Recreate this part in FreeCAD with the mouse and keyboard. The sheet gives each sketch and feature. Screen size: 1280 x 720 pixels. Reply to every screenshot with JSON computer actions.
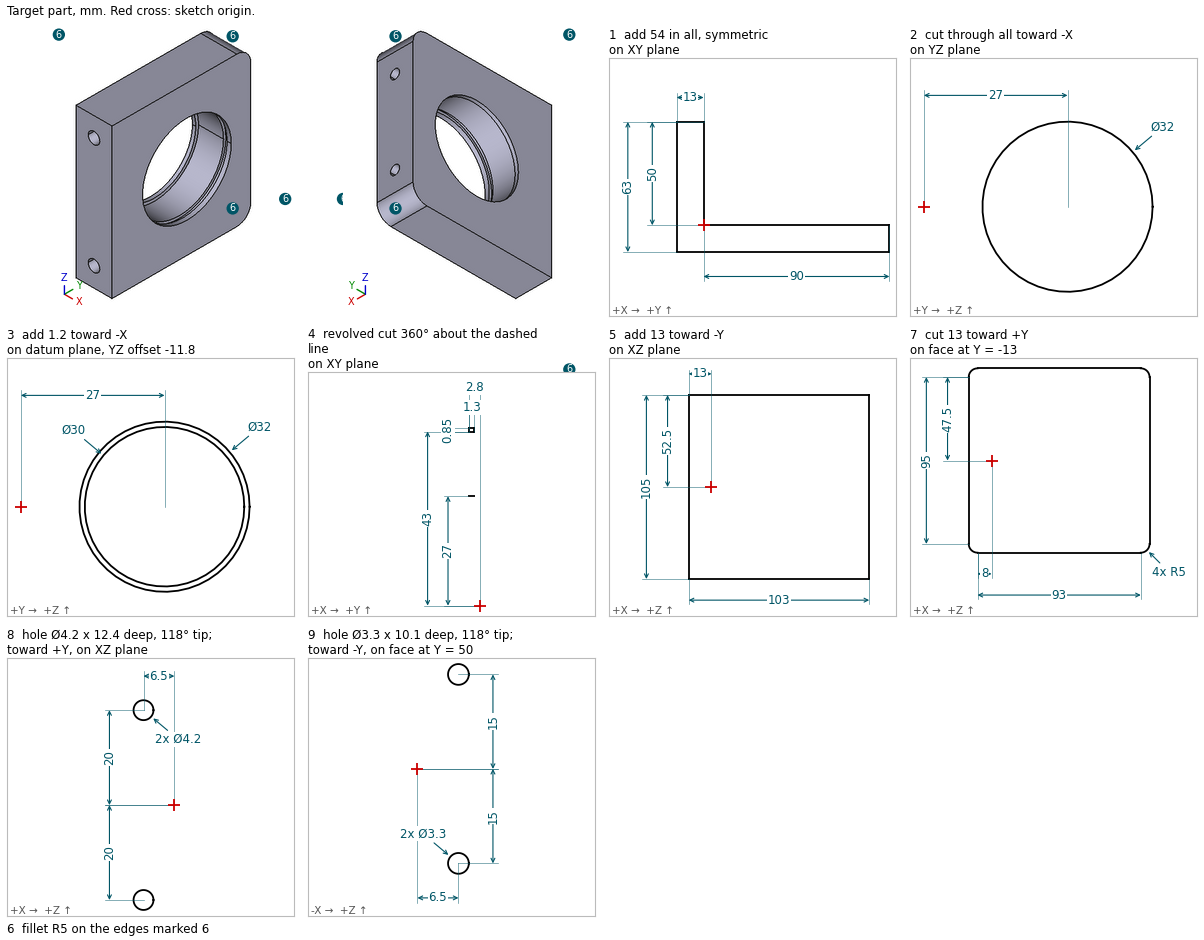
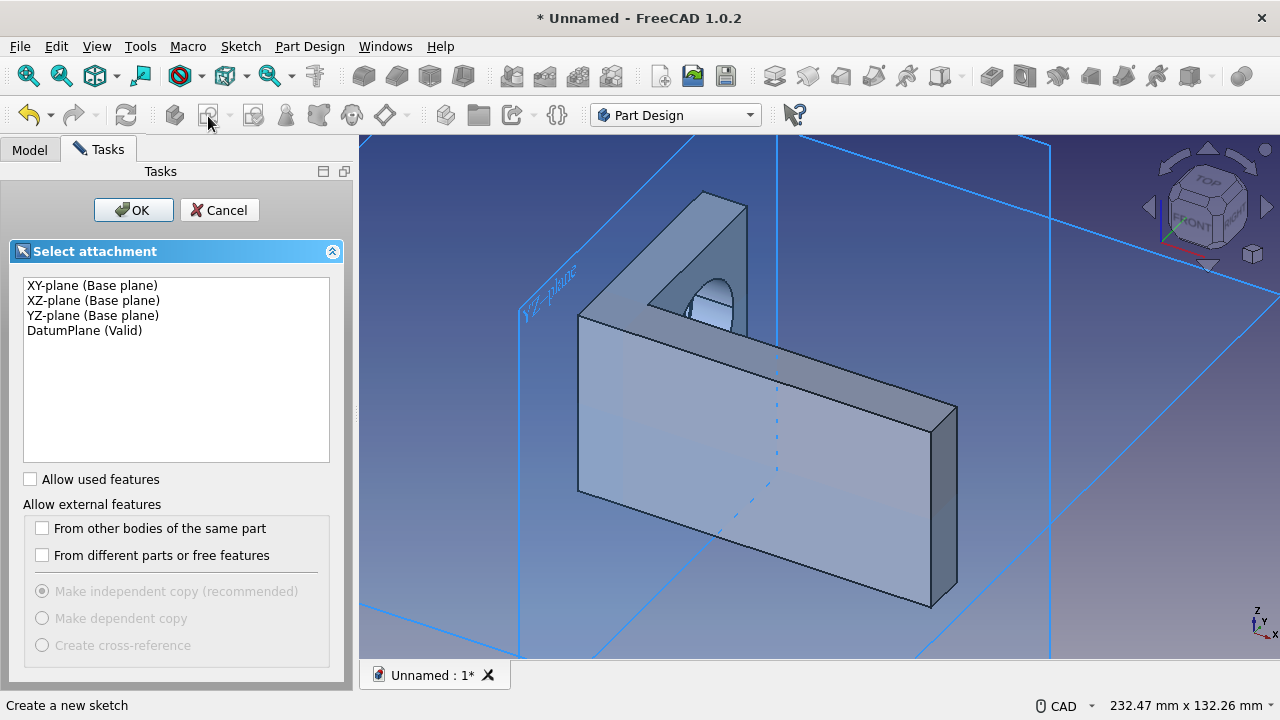
{"action": "left_click", "coordinate": [84, 286]}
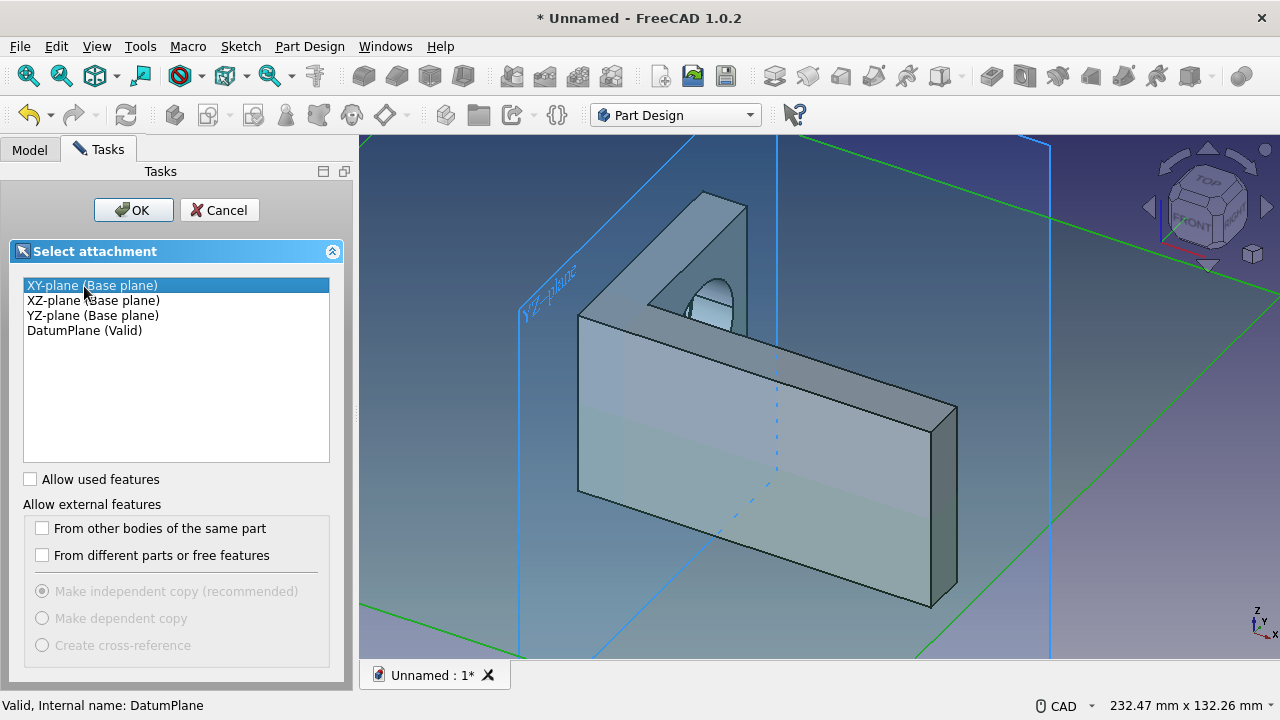
{"action": "left_click", "coordinate": [134, 210]}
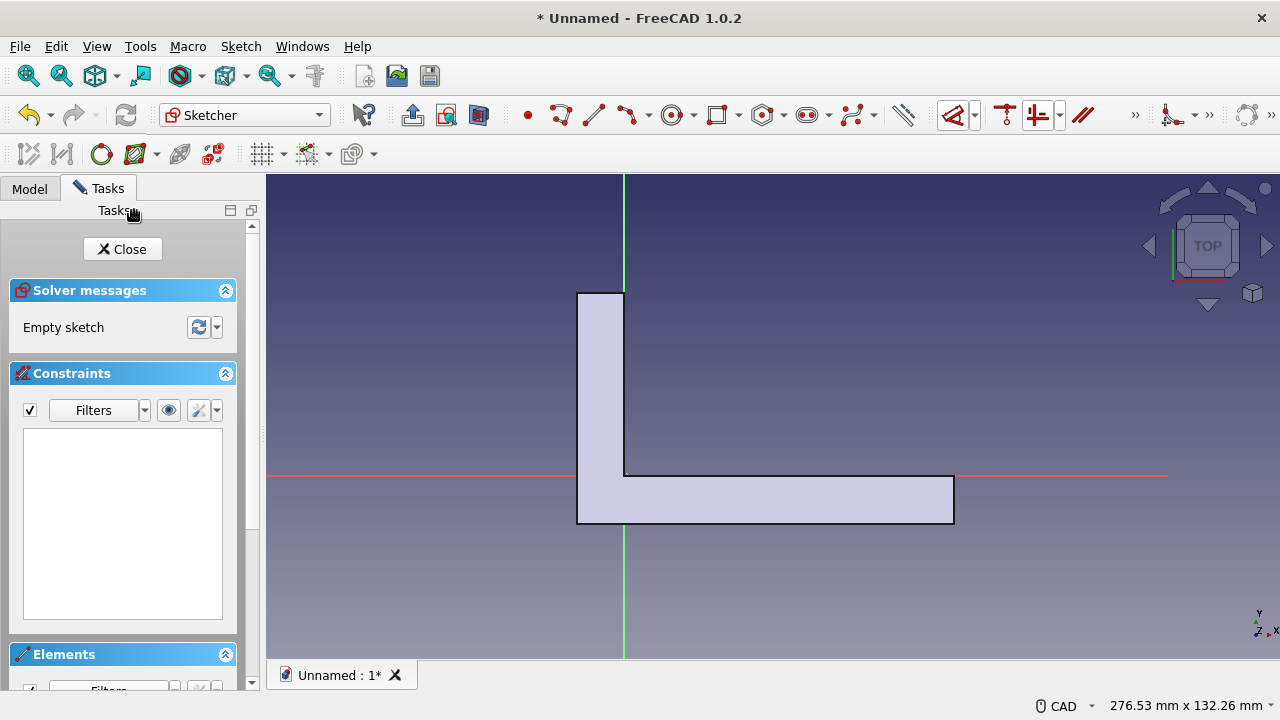
{"action": "left_click", "coordinate": [479, 116]}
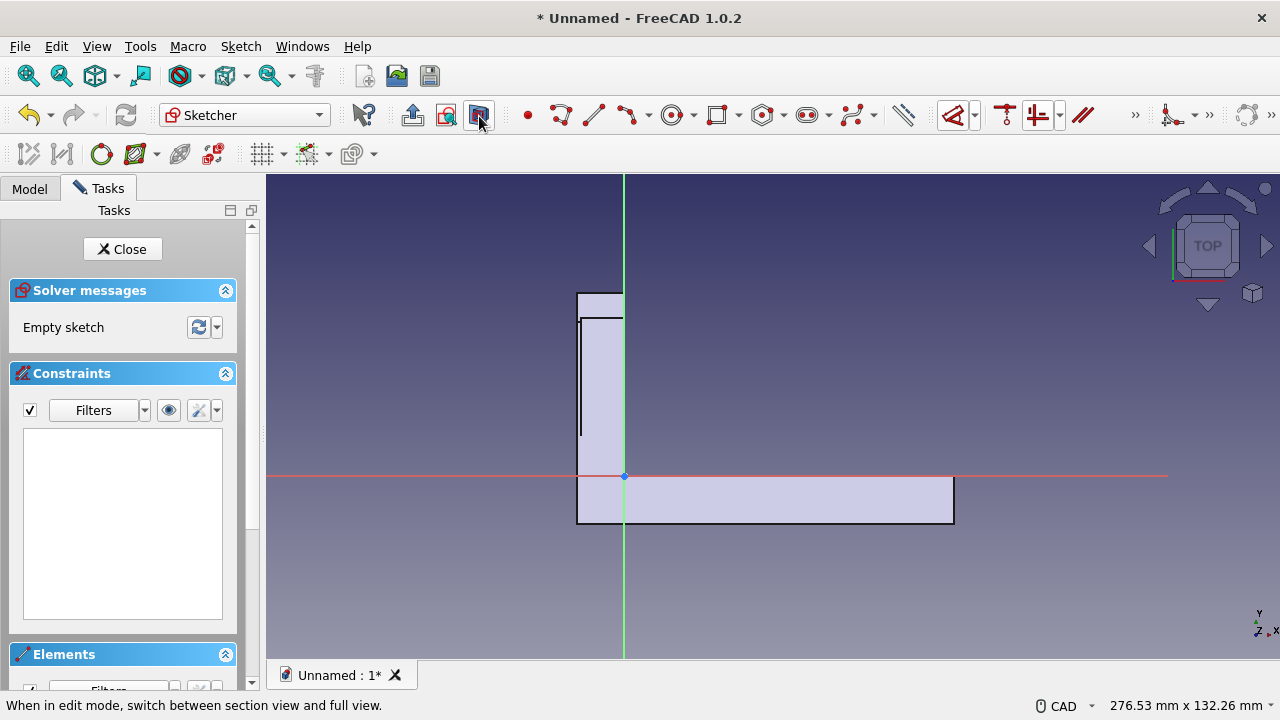
{"action": "scroll", "coordinate": [594, 328], "scroll_direction": "up", "scroll_amount": 8}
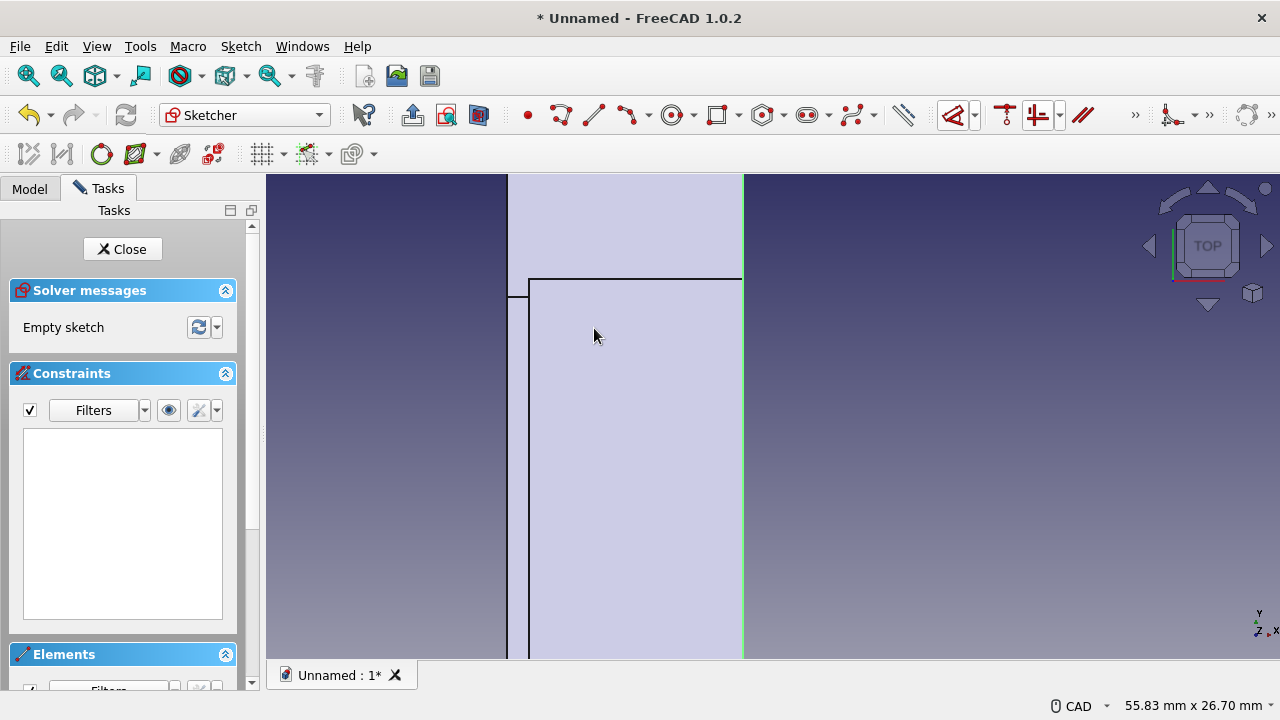
{"action": "left_click", "coordinate": [716, 116]}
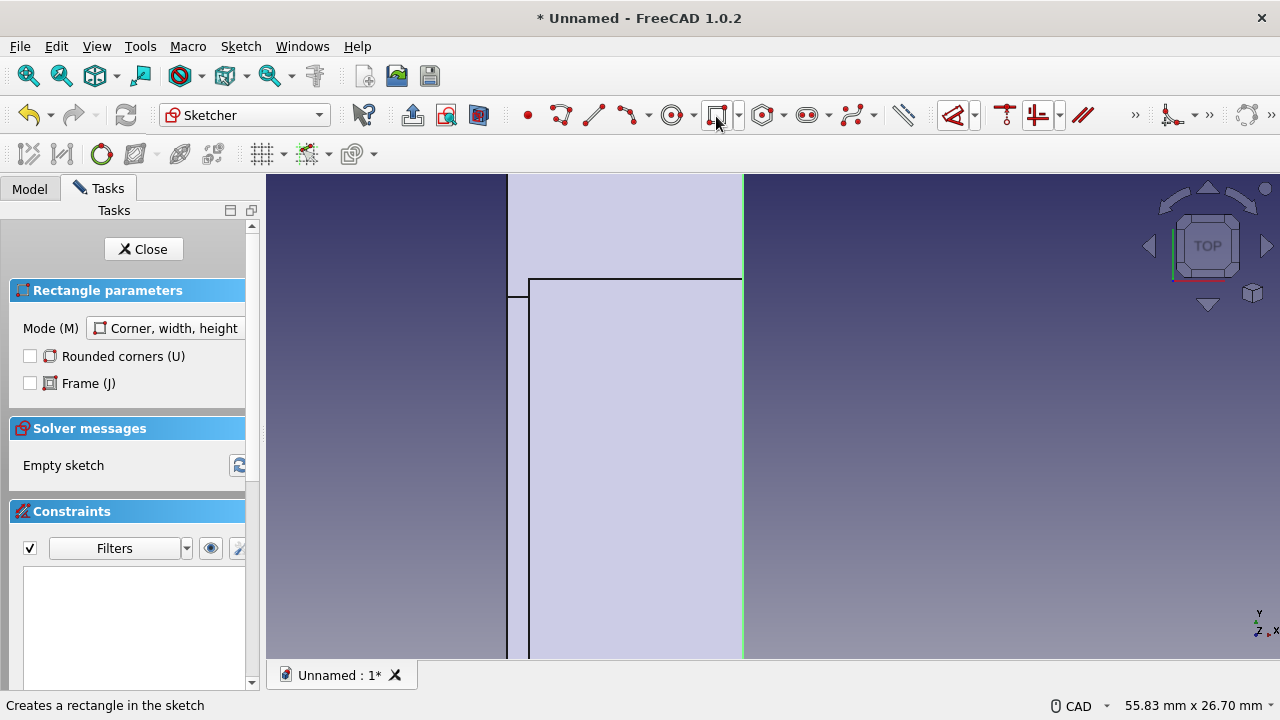
{"action": "left_click", "coordinate": [692, 264]}
{"action": "left_click", "coordinate": [716, 279]}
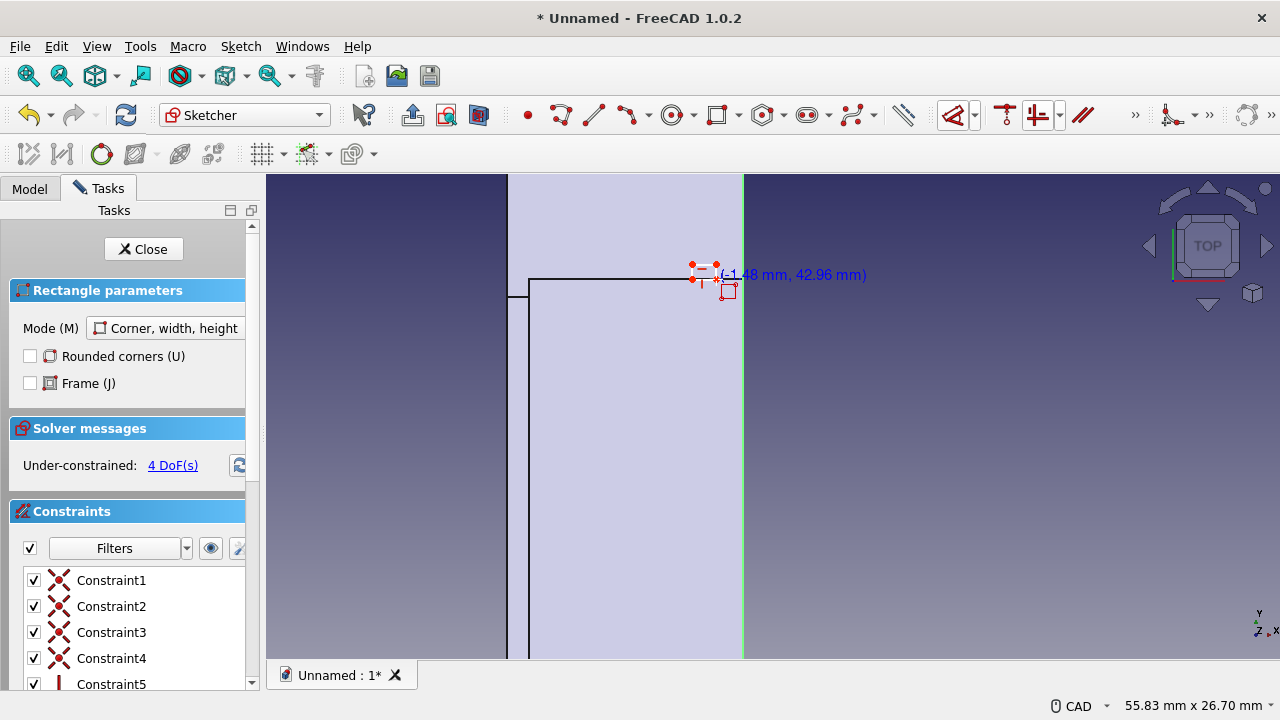
{"action": "left_click", "coordinate": [594, 116]}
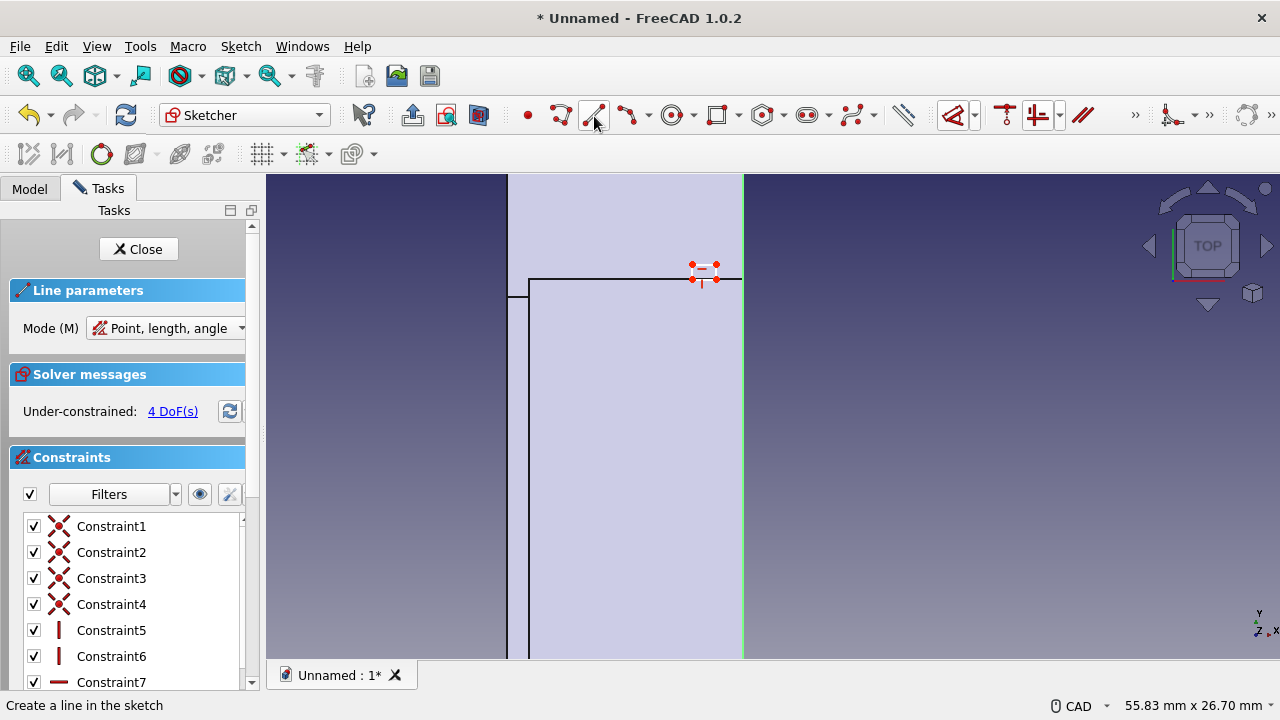
{"action": "left_click", "coordinate": [690, 570]}
{"action": "left_click", "coordinate": [718, 570]}
{"action": "key", "text": "Escape"}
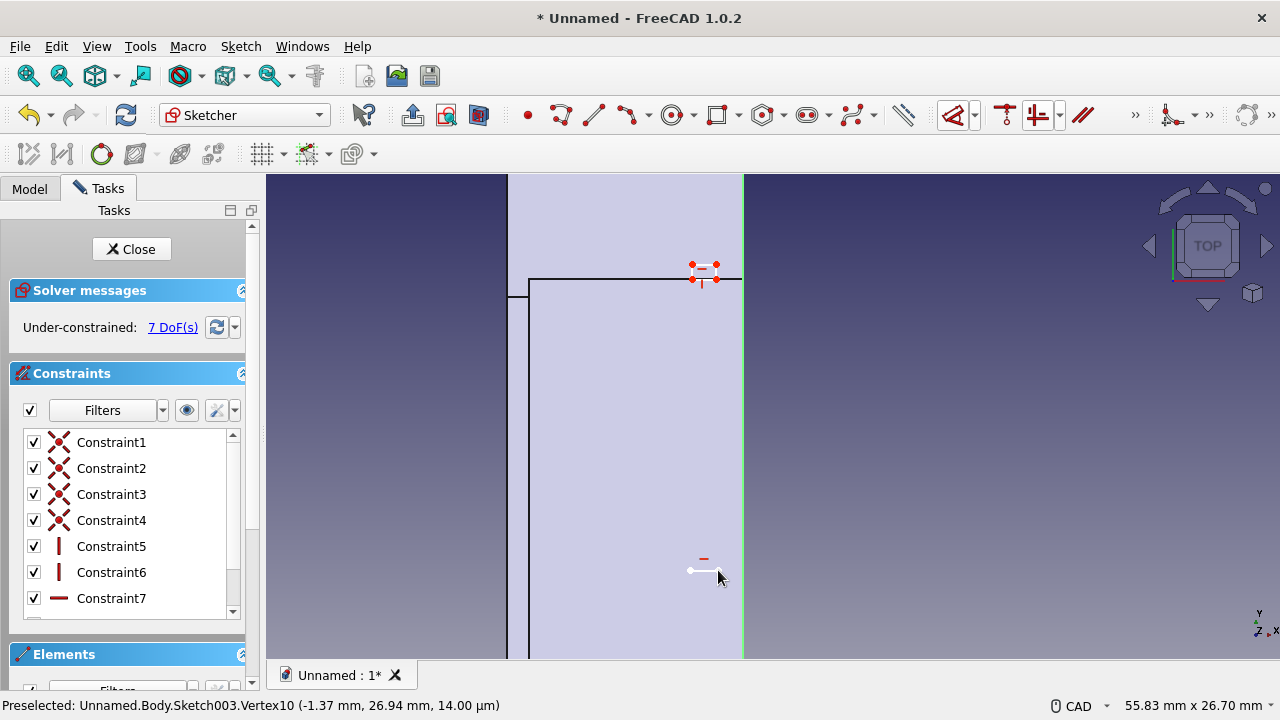
{"action": "scroll", "coordinate": [701, 571], "scroll_direction": "up", "scroll_amount": 2}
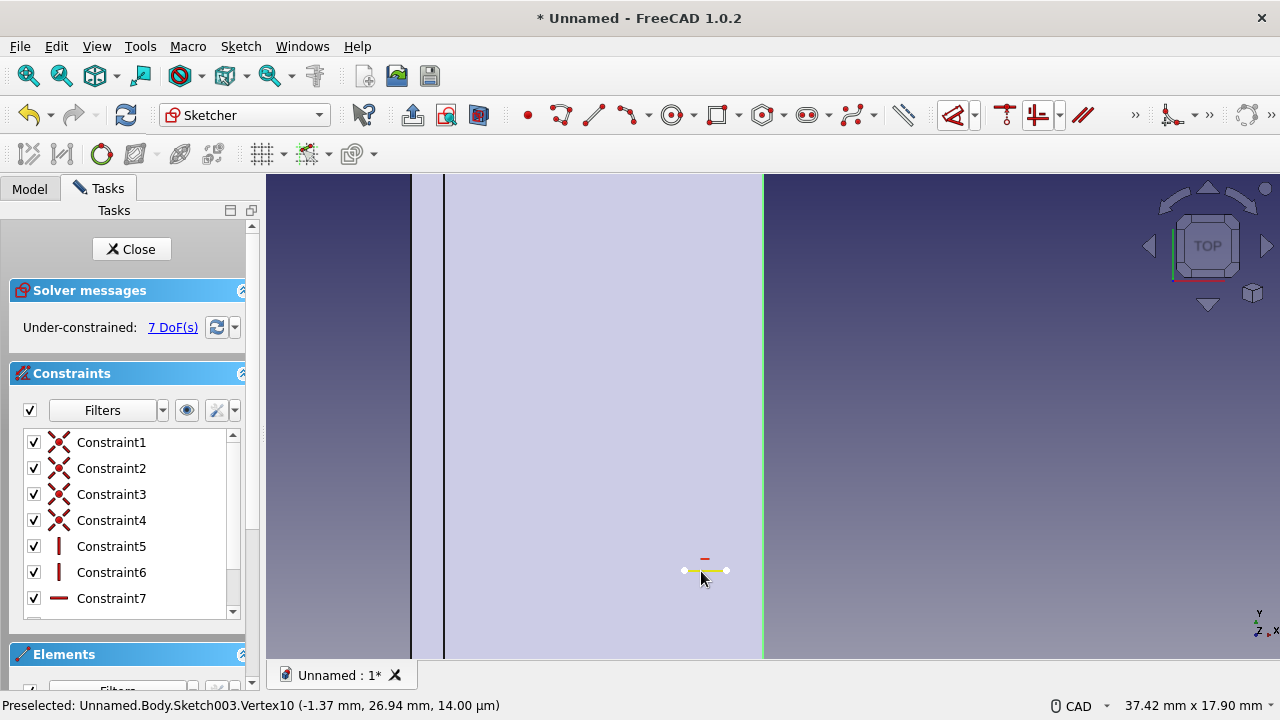
{"action": "left_click", "coordinate": [701, 571]}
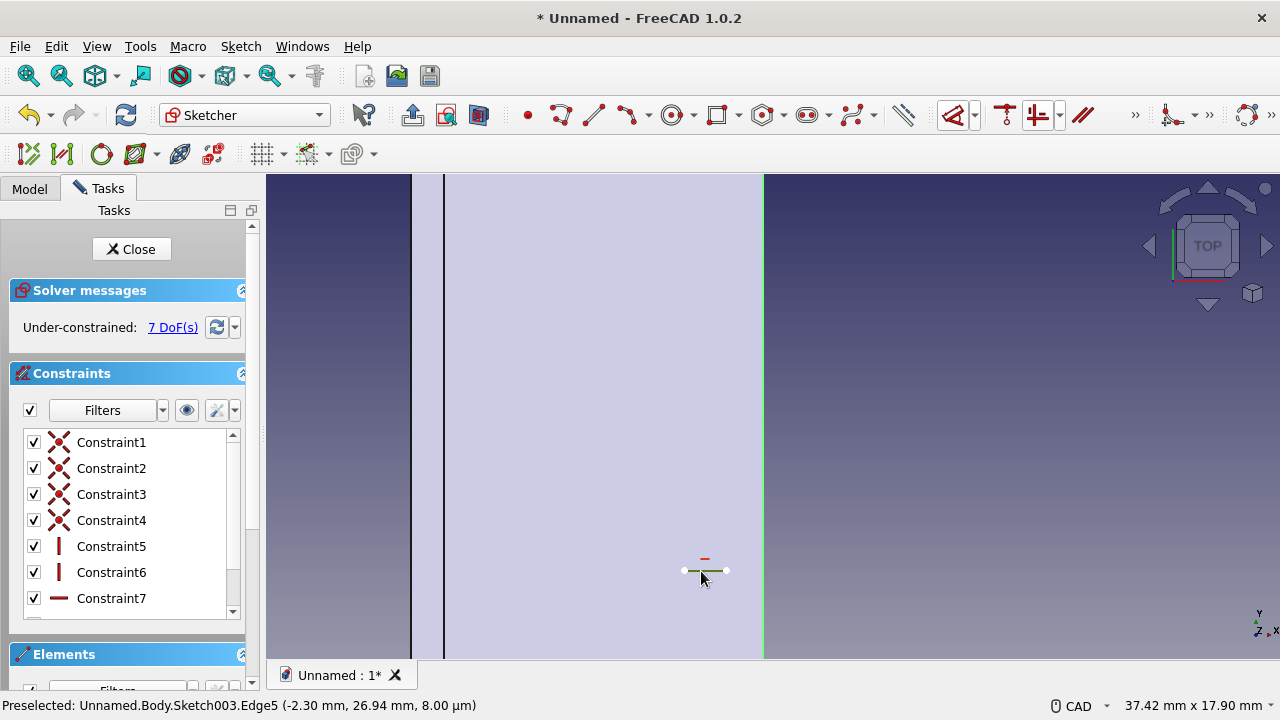
{"action": "left_click", "coordinate": [904, 116]}